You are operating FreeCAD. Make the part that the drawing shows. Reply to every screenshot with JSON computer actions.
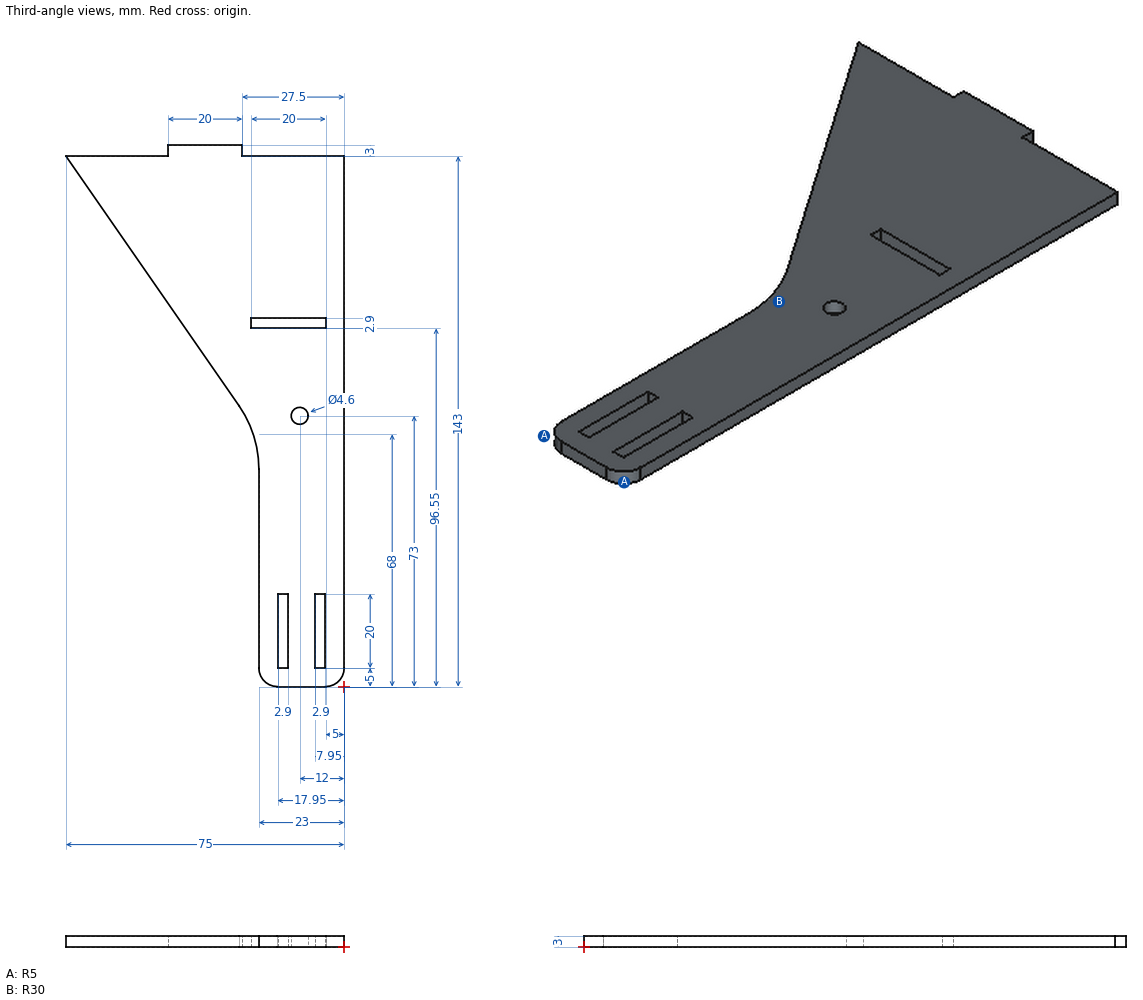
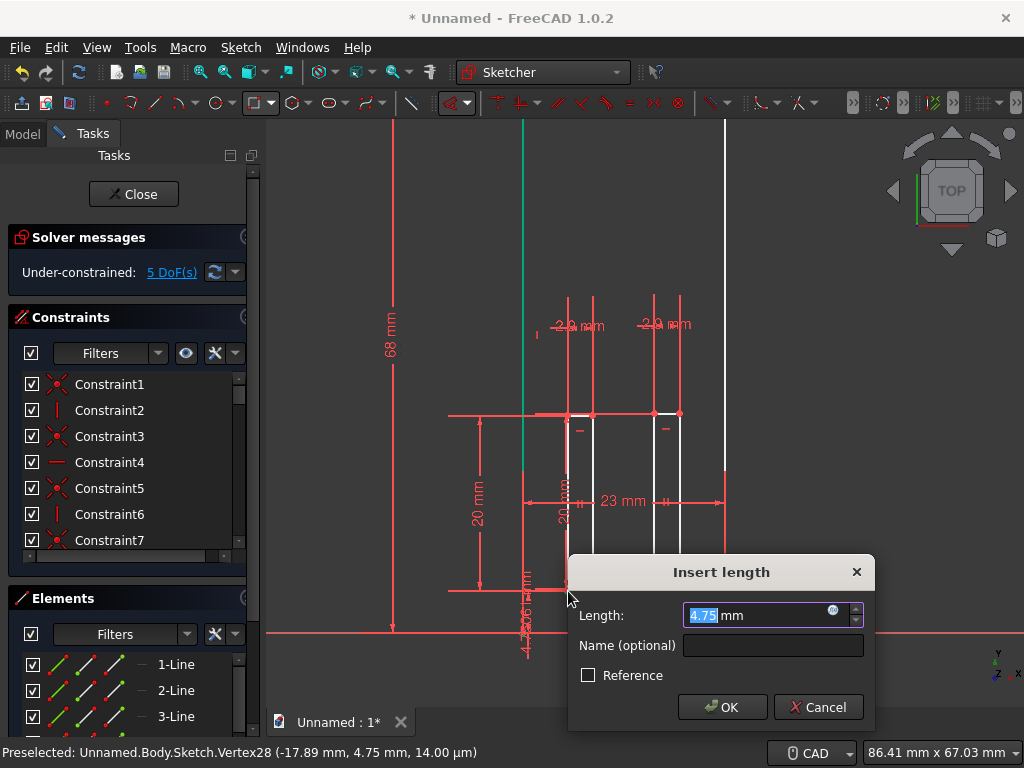
{"action": "type", "text": "5"}
{"action": "key", "text": "Return"}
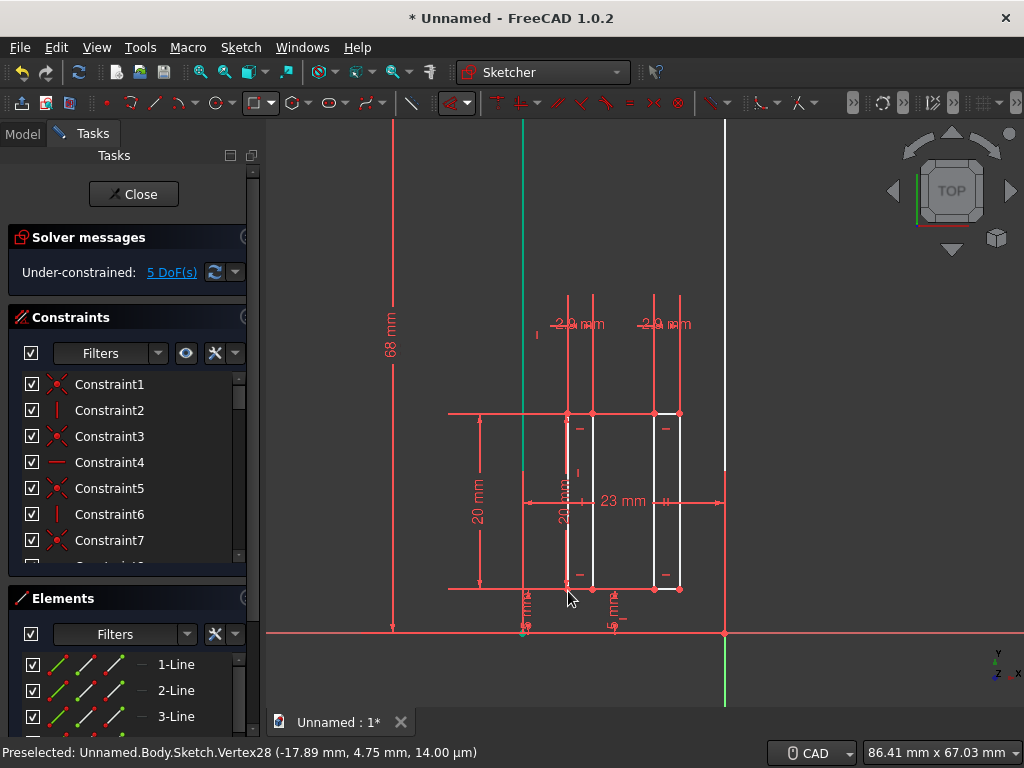
{"action": "left_click", "coordinate": [725, 257]}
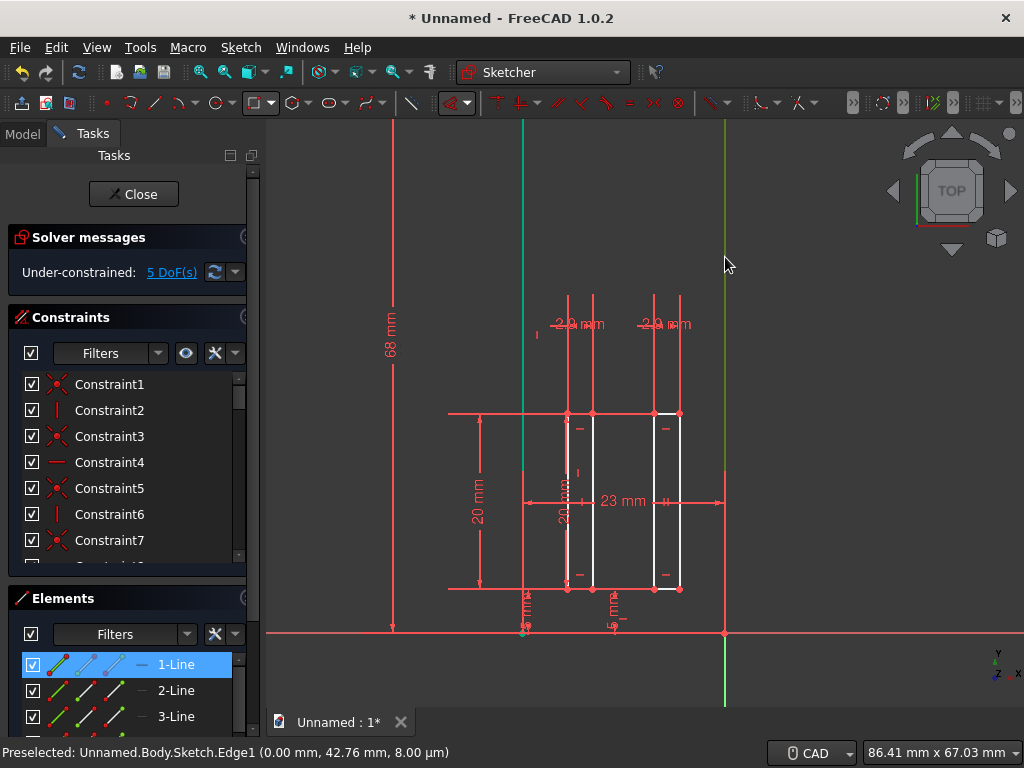
{"action": "left_click", "coordinate": [470, 104]}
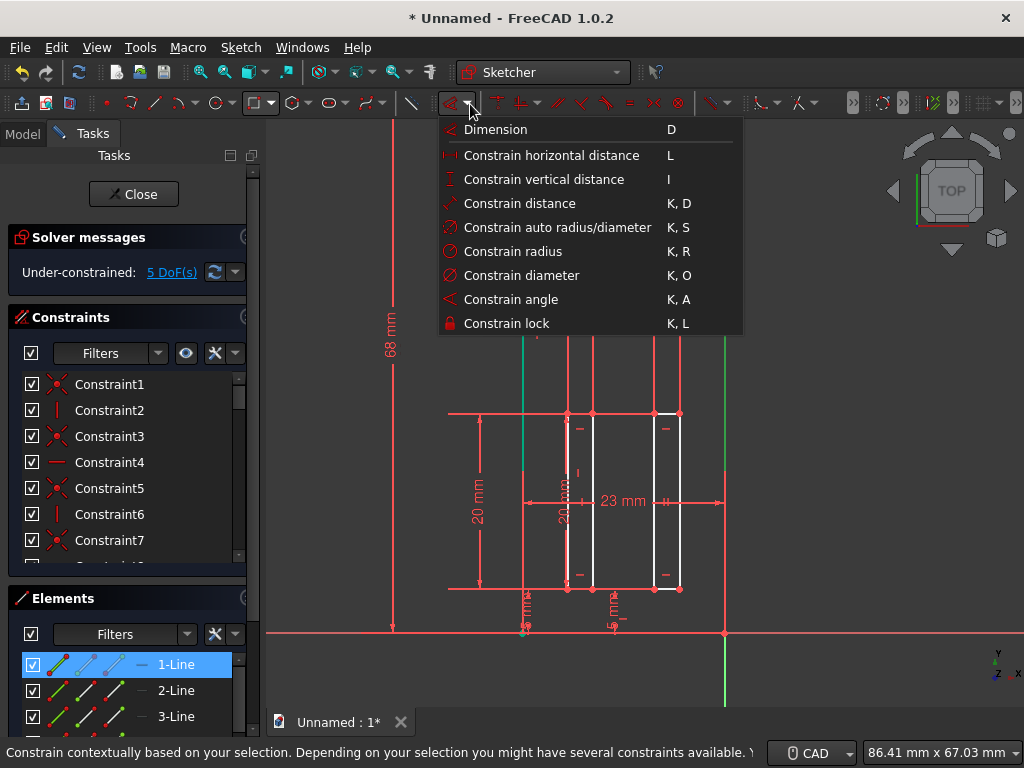
{"action": "left_click", "coordinate": [591, 179]}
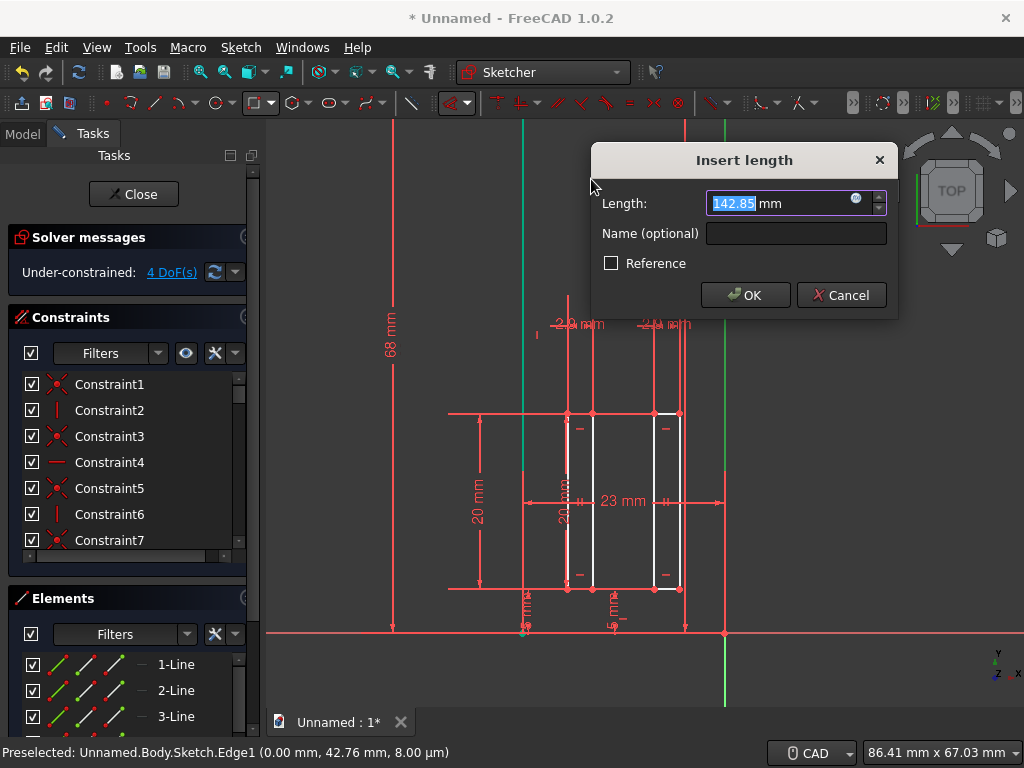
{"action": "type", "text": "143"}
{"action": "key", "text": "Return"}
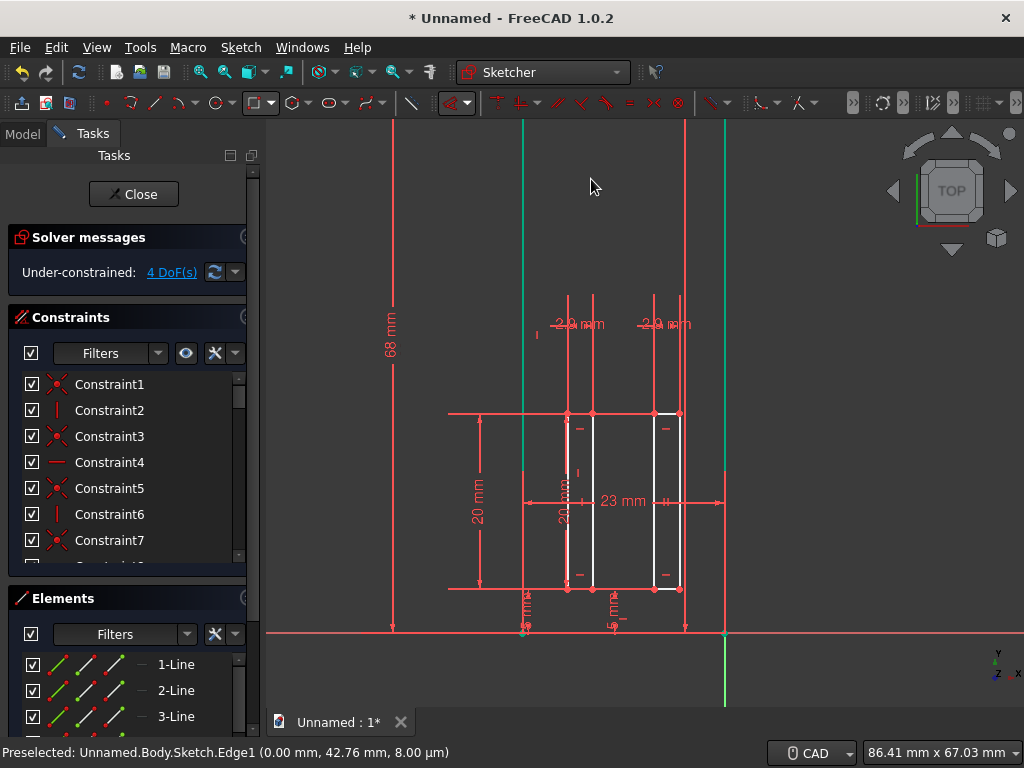
{"action": "scroll", "coordinate": [654, 594], "scroll_direction": "down", "scroll_amount": 6}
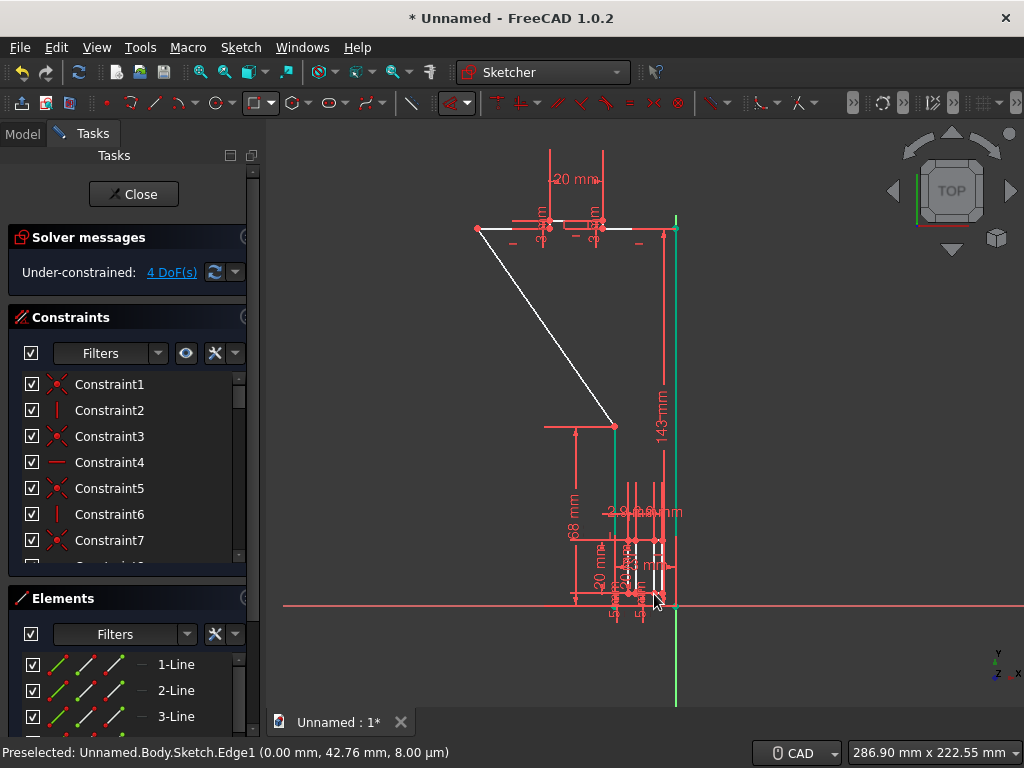
{"action": "left_click", "coordinate": [477, 229]}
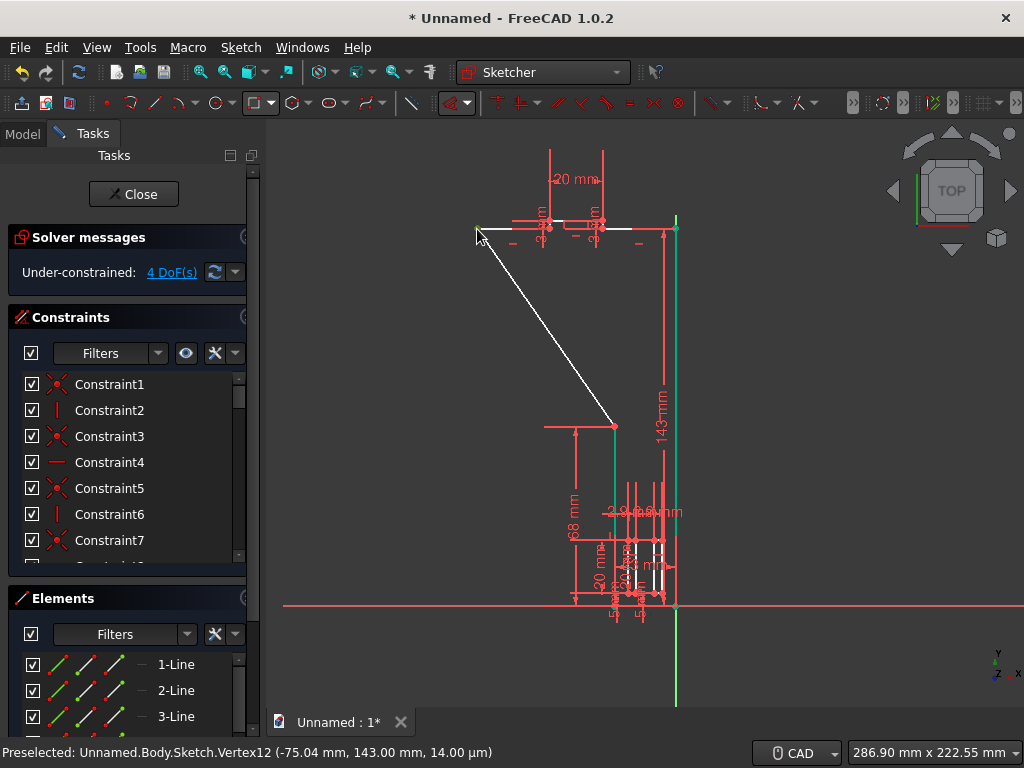
{"action": "left_click", "coordinate": [470, 104]}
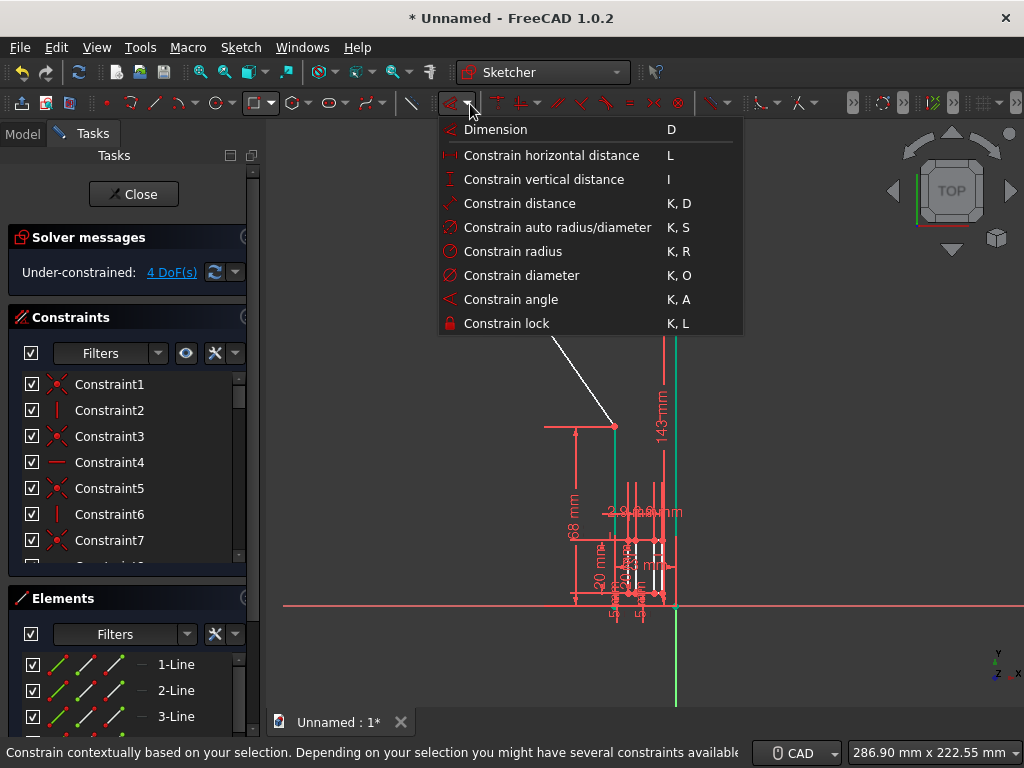
{"action": "left_click", "coordinate": [591, 155]}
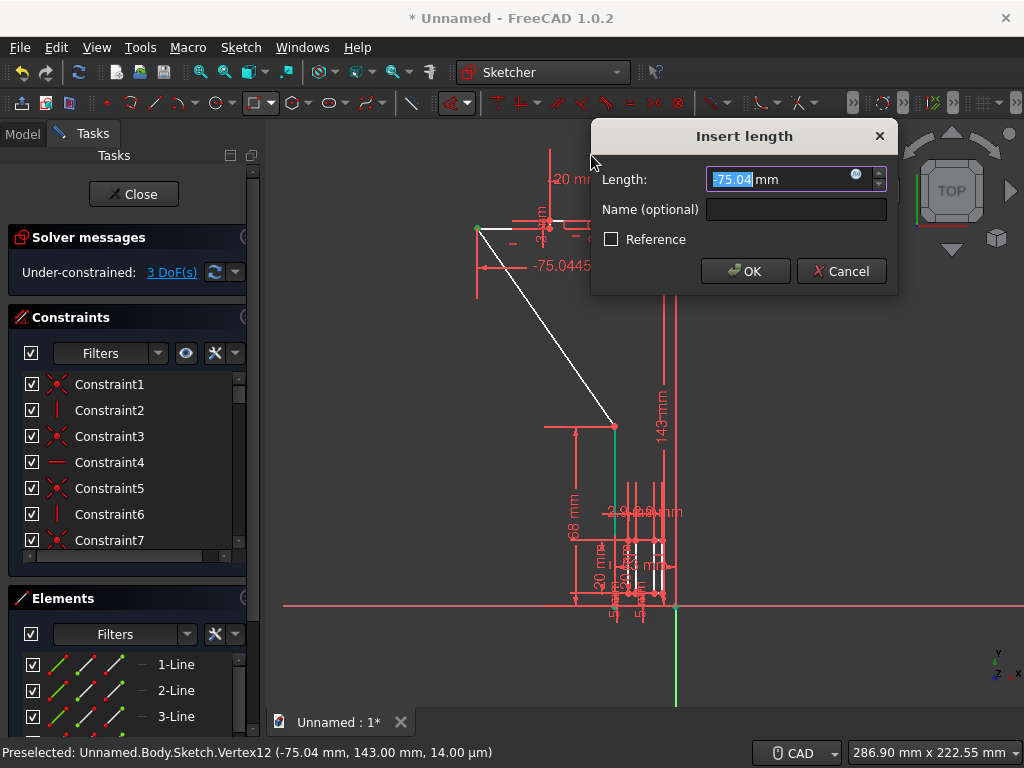
{"action": "type", "text": "-75"}
{"action": "key", "text": "Return"}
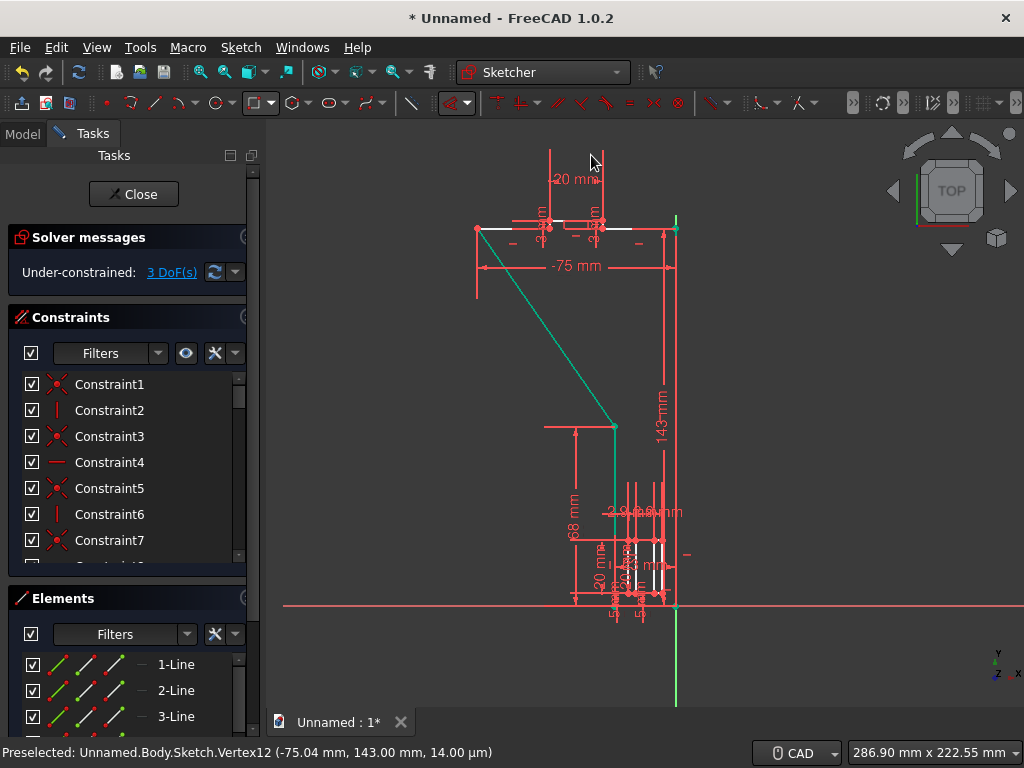
{"action": "left_click", "coordinate": [654, 229]}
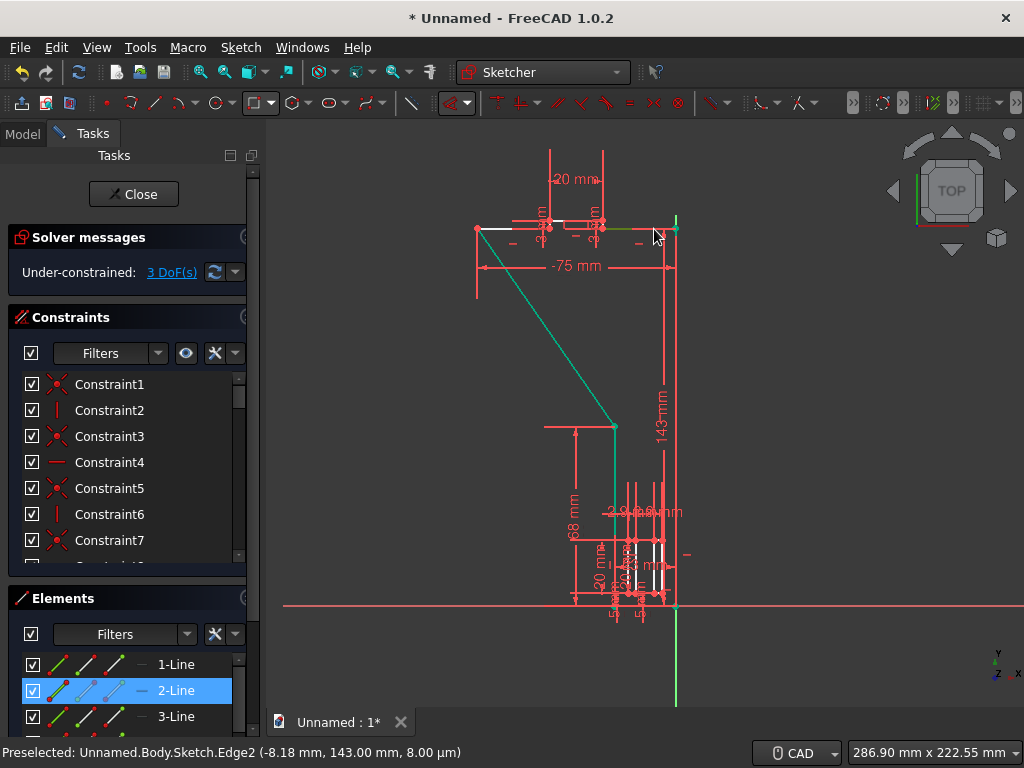
{"action": "key", "text": "l"}